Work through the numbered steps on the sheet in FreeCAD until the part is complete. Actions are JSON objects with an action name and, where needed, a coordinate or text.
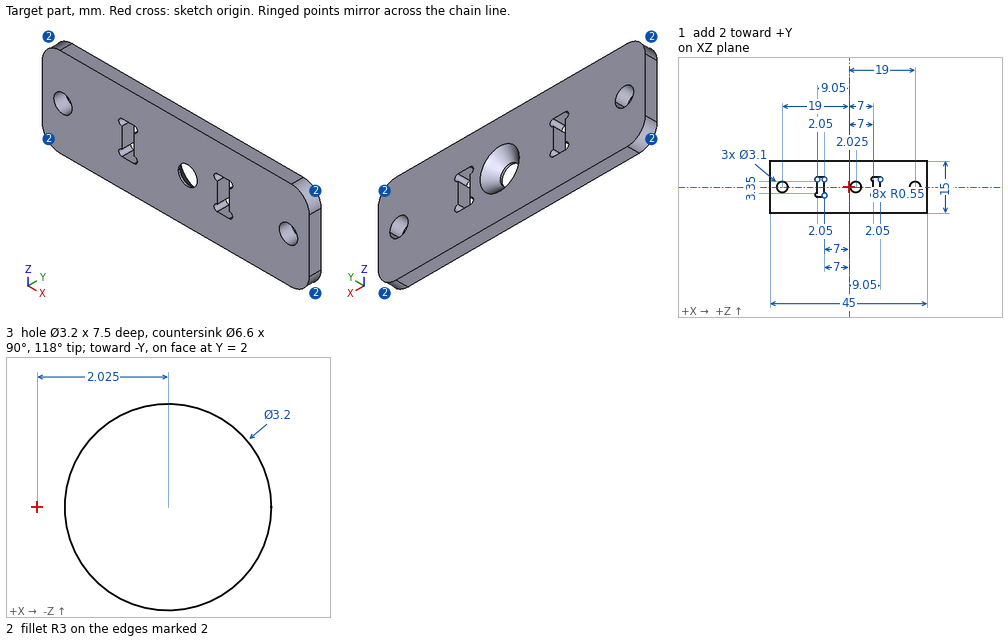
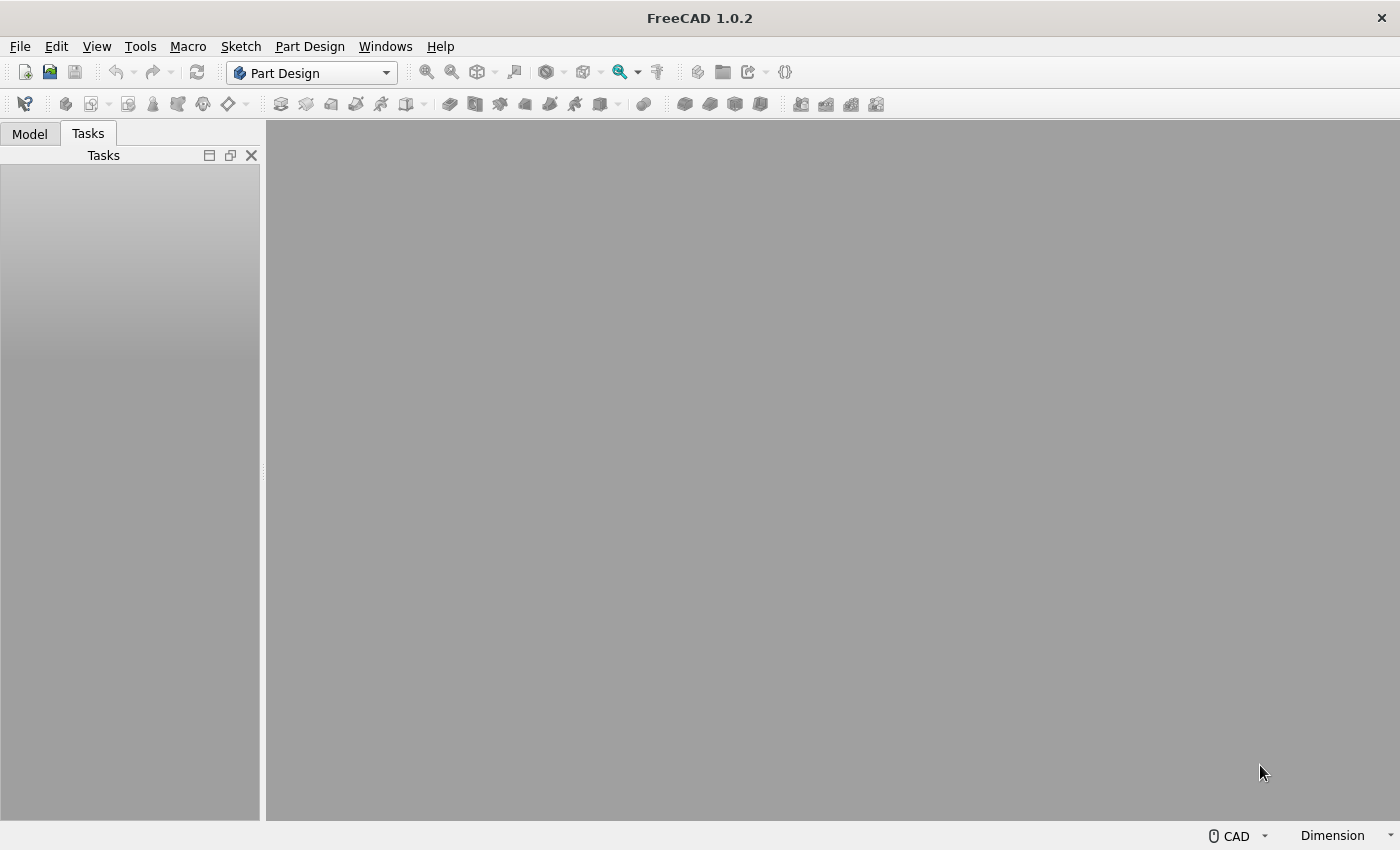
{"action": "left_click", "coordinate": [25, 72]}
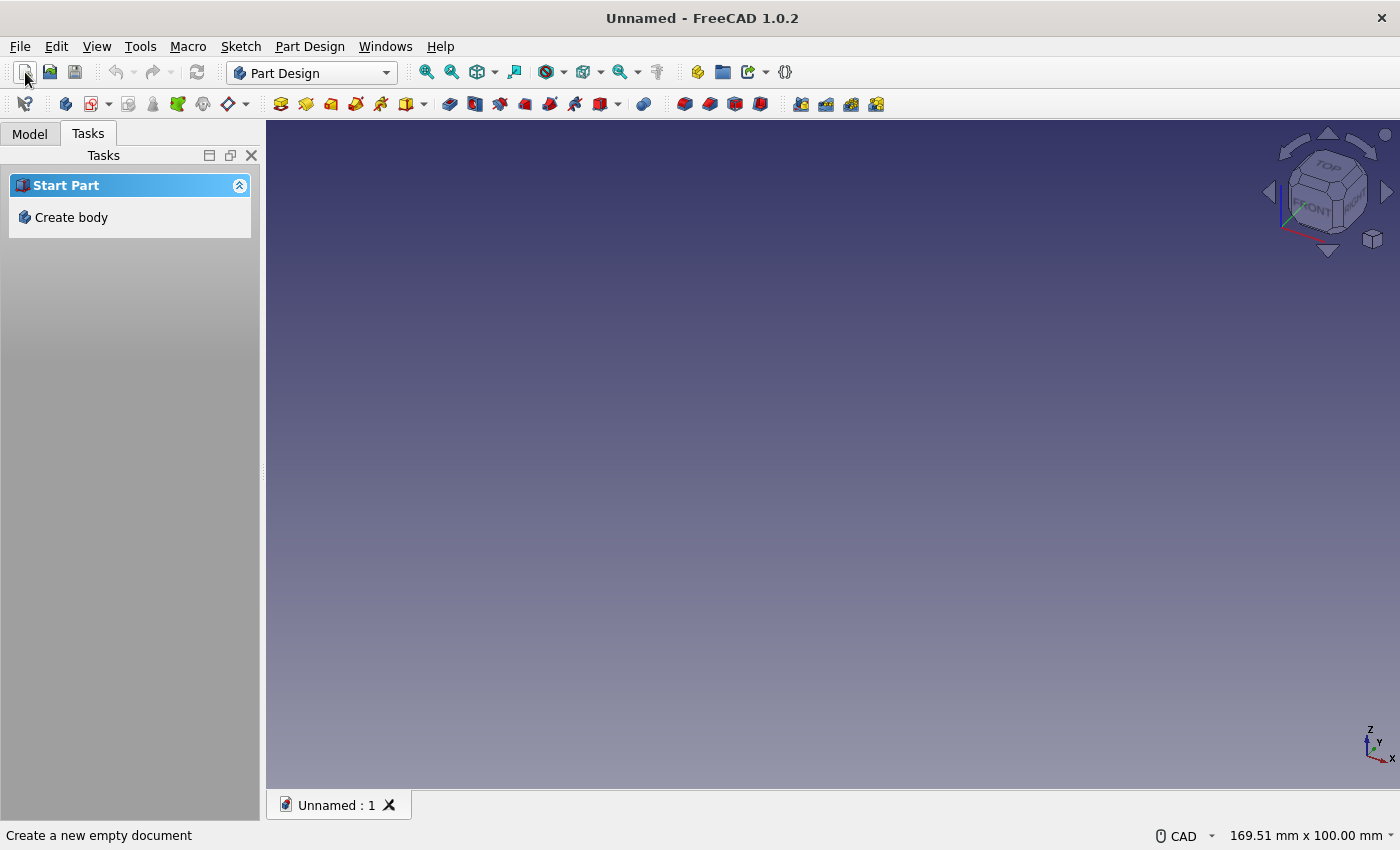
{"action": "left_click", "coordinate": [90, 104]}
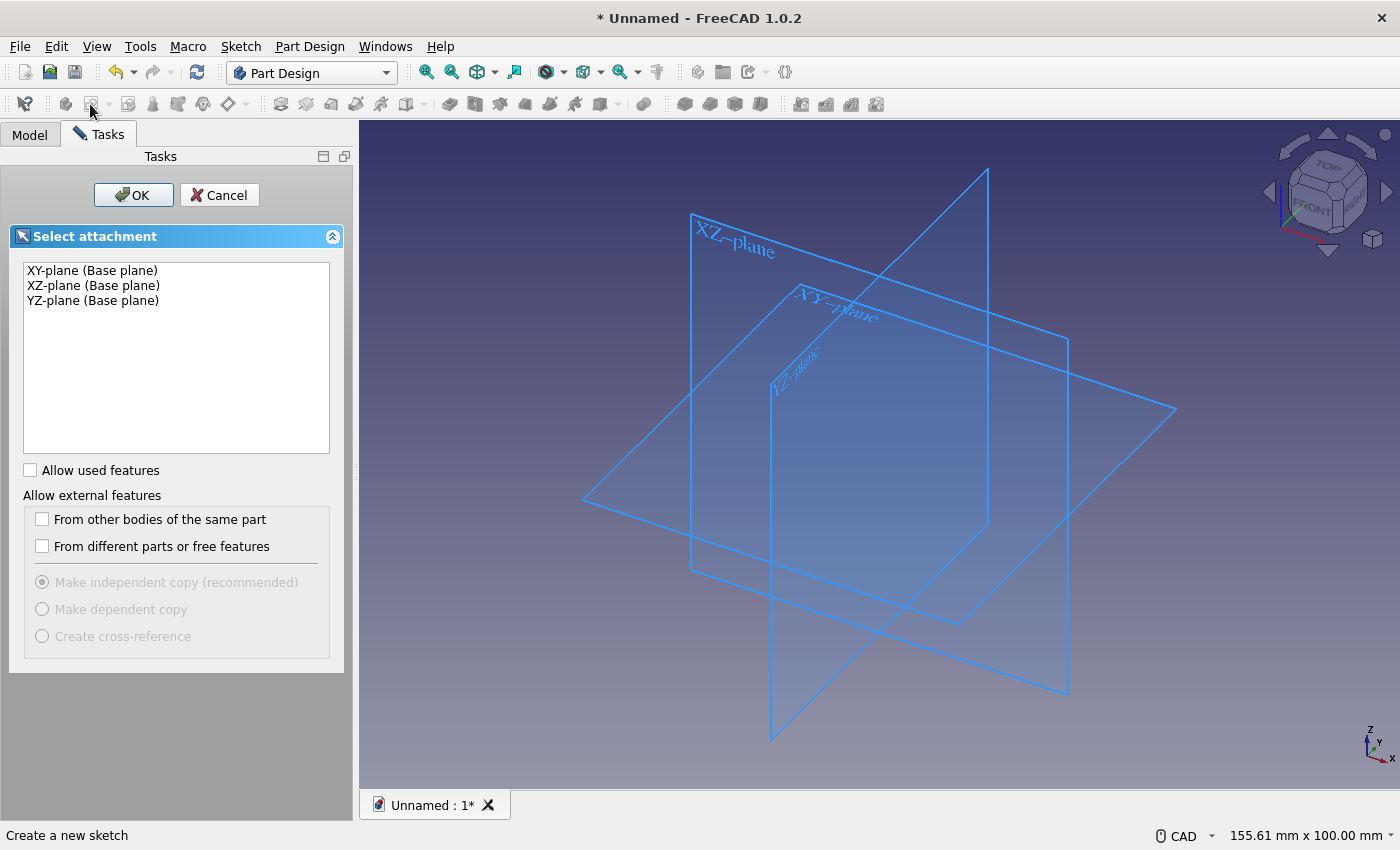
{"action": "left_click", "coordinate": [84, 286]}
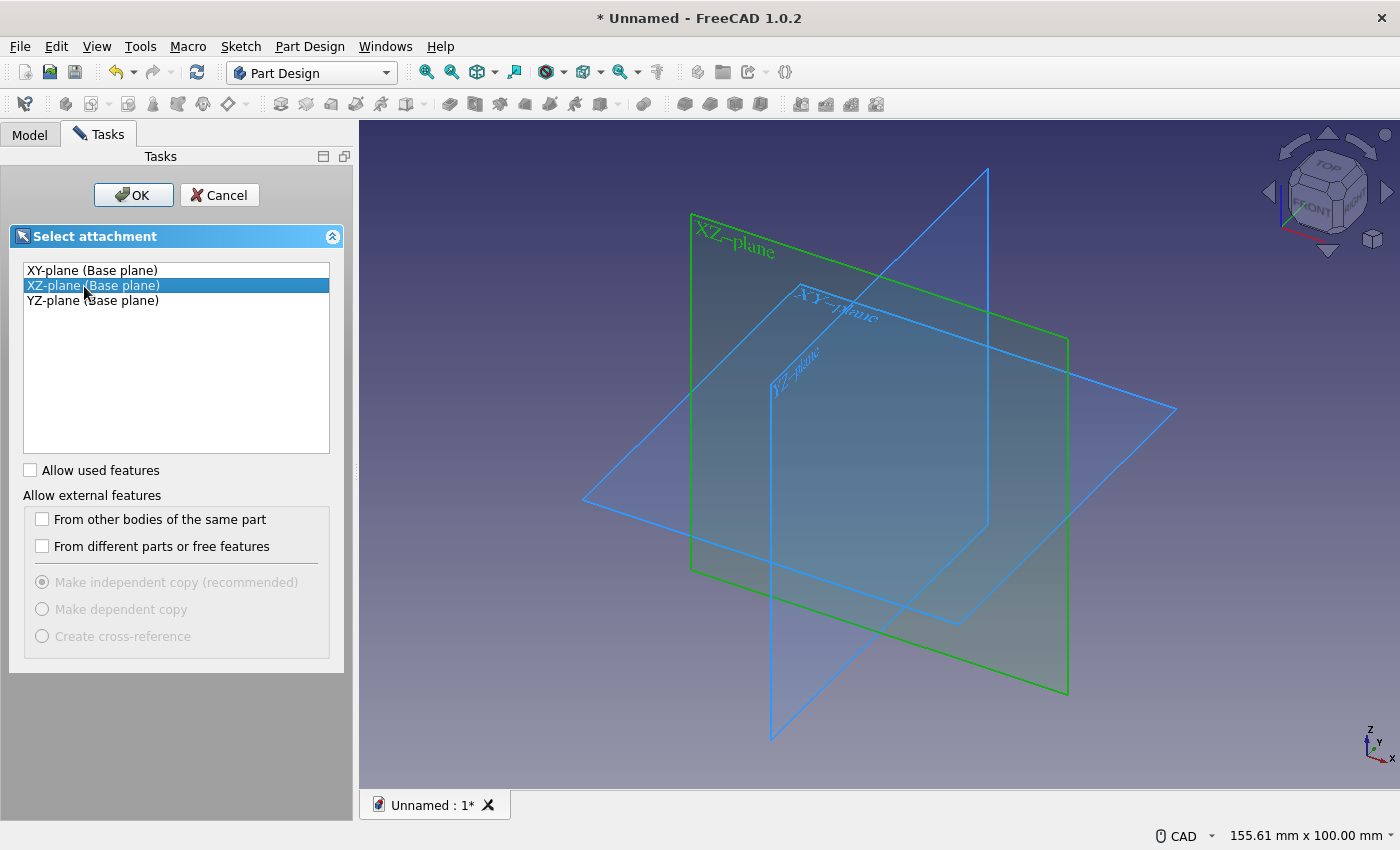
{"action": "left_click", "coordinate": [134, 195]}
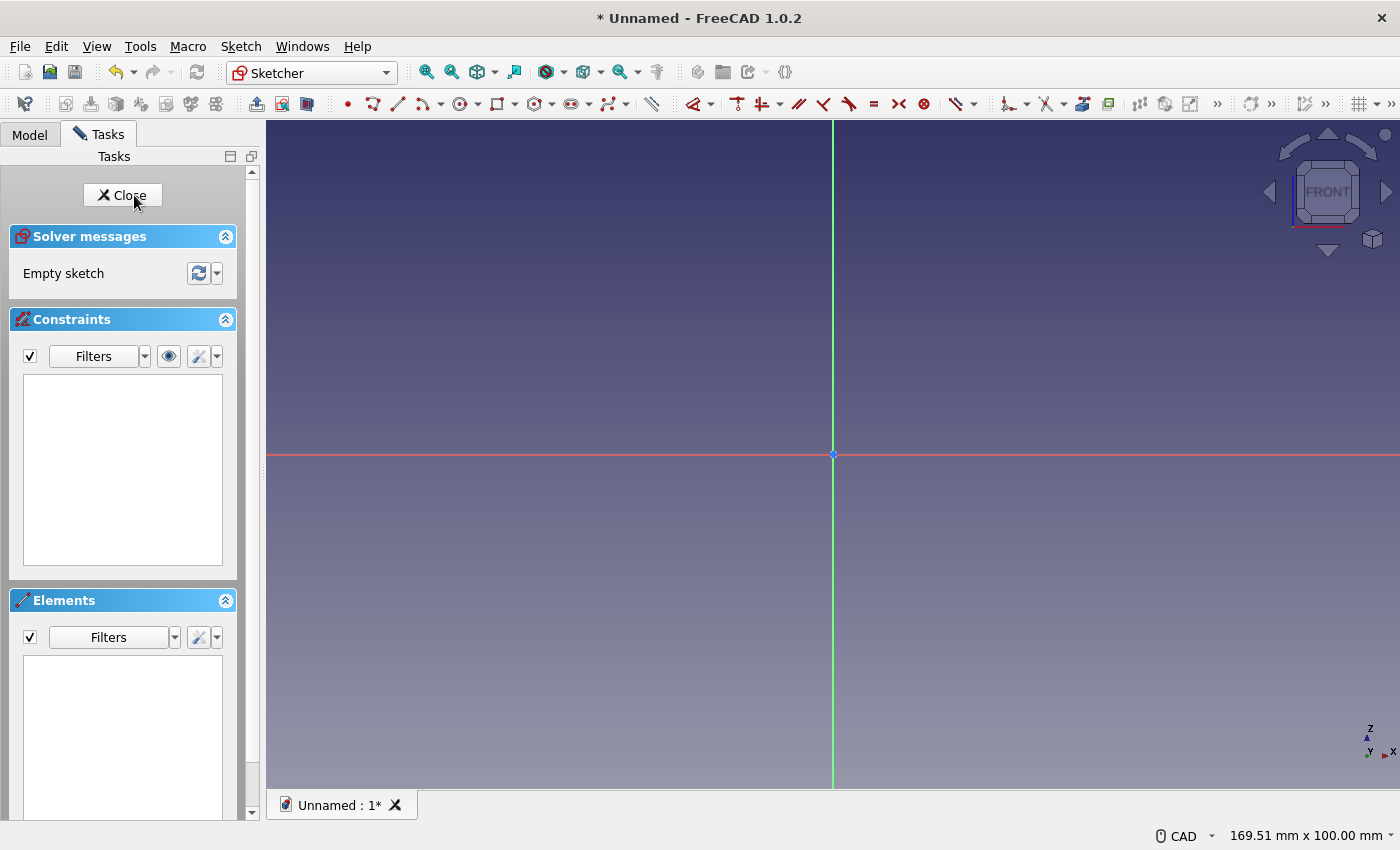
{"action": "scroll", "coordinate": [889, 455], "scroll_direction": "up", "scroll_amount": 4}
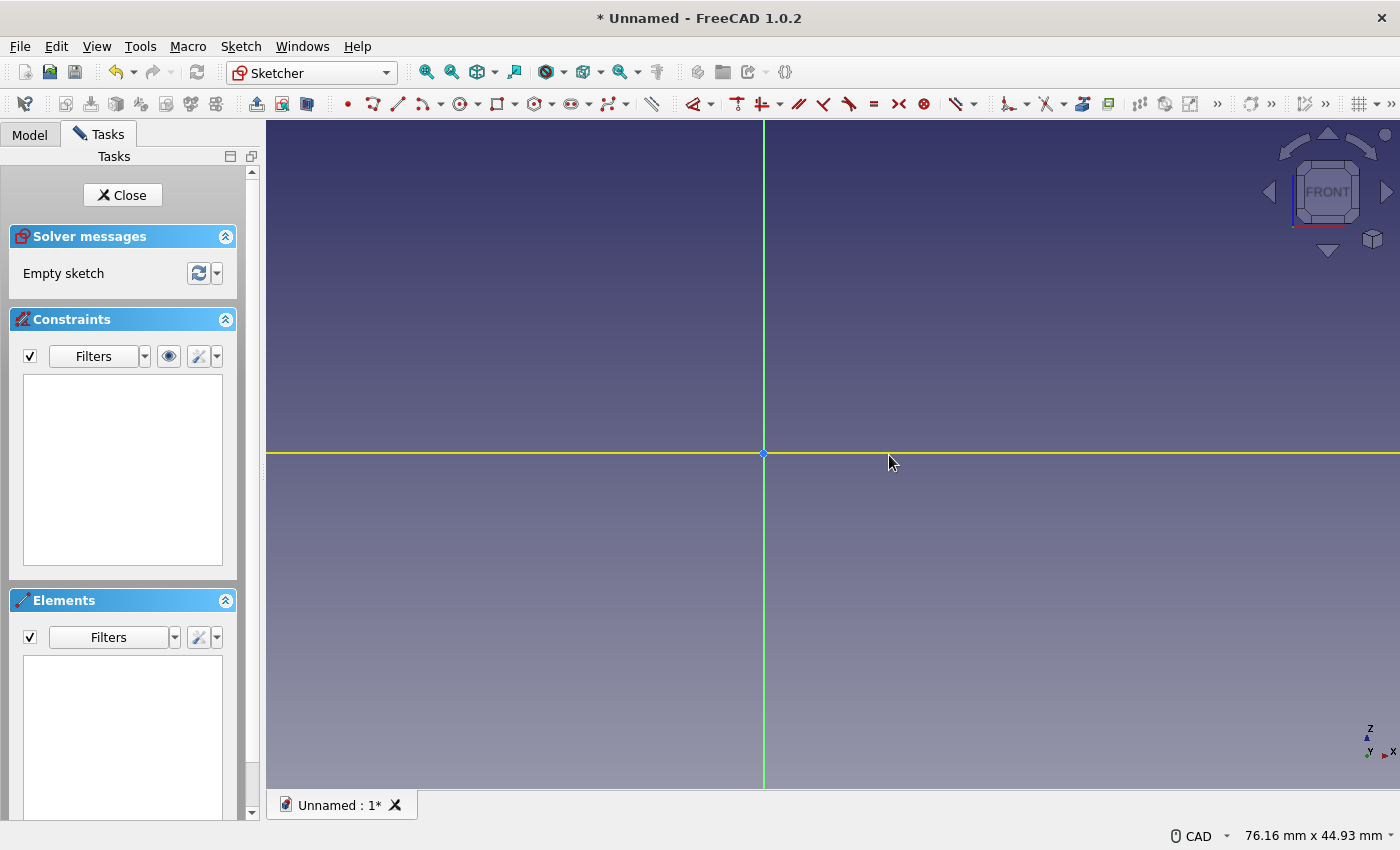
{"action": "key", "text": "g v"}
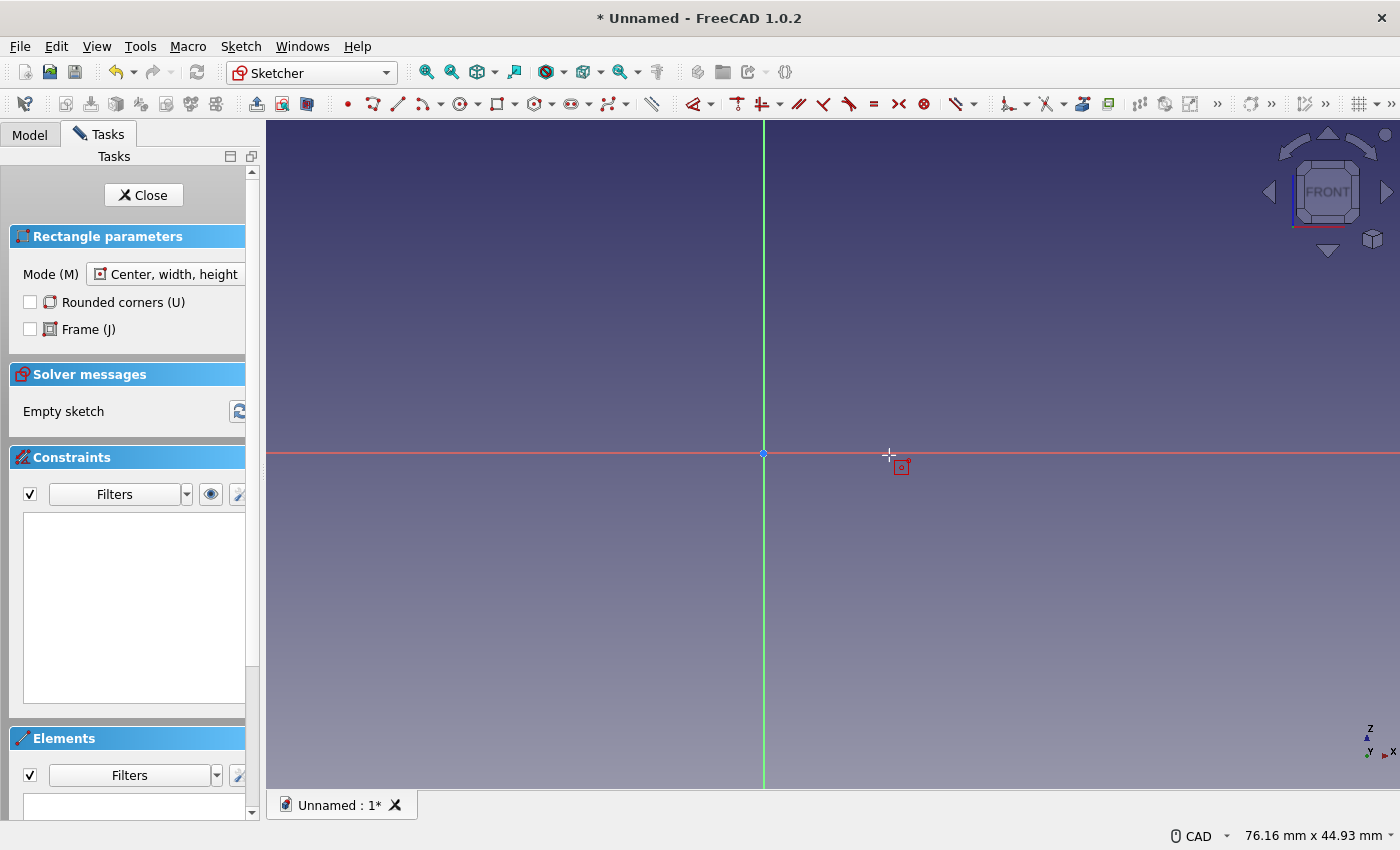
{"action": "left_click", "coordinate": [764, 453]}
{"action": "mouse_move", "coordinate": [1099, 342]}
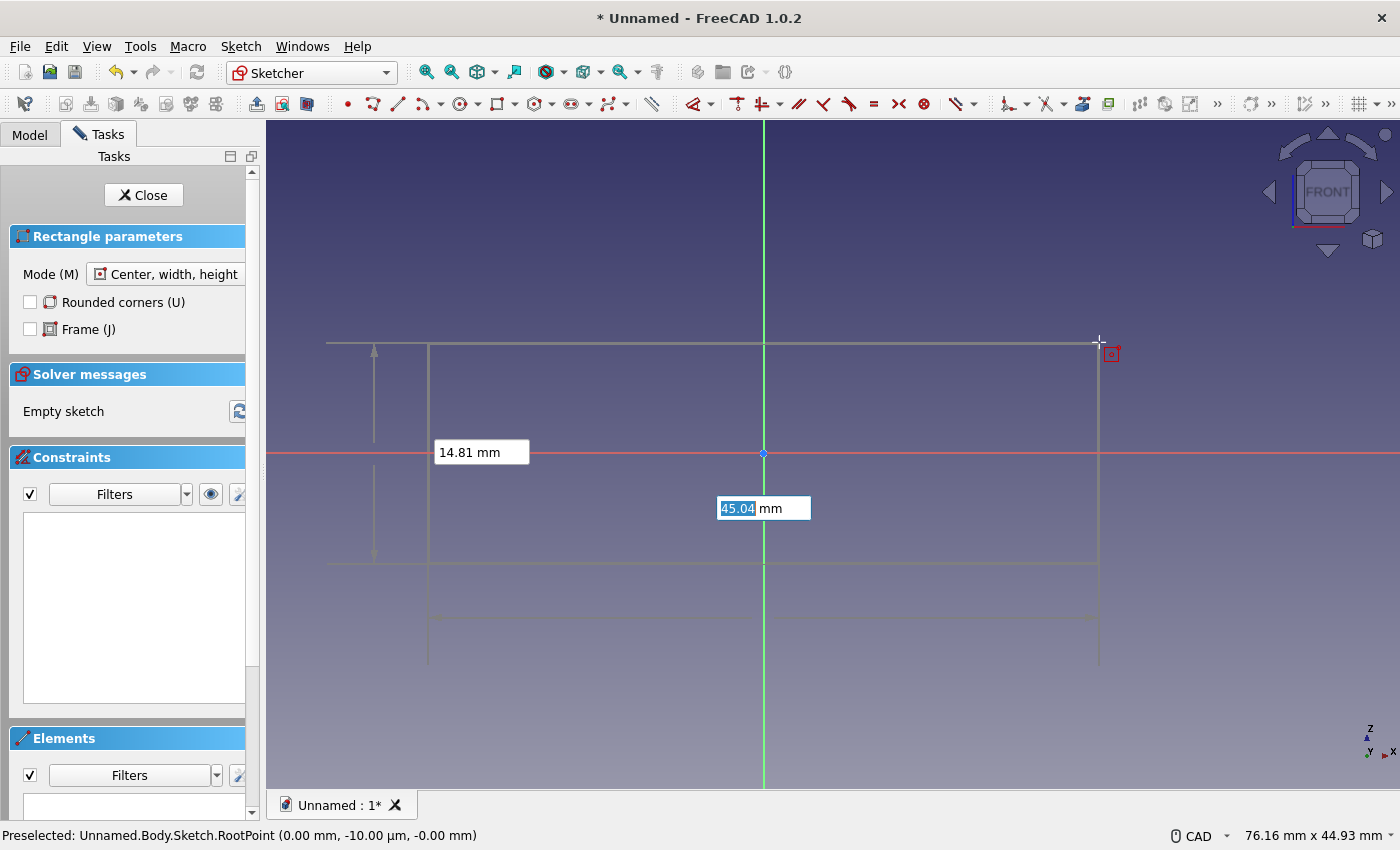
{"action": "type", "text": "45"}
{"action": "key", "text": "Tab"}
{"action": "type", "text": "15"}
{"action": "key", "text": "Return"}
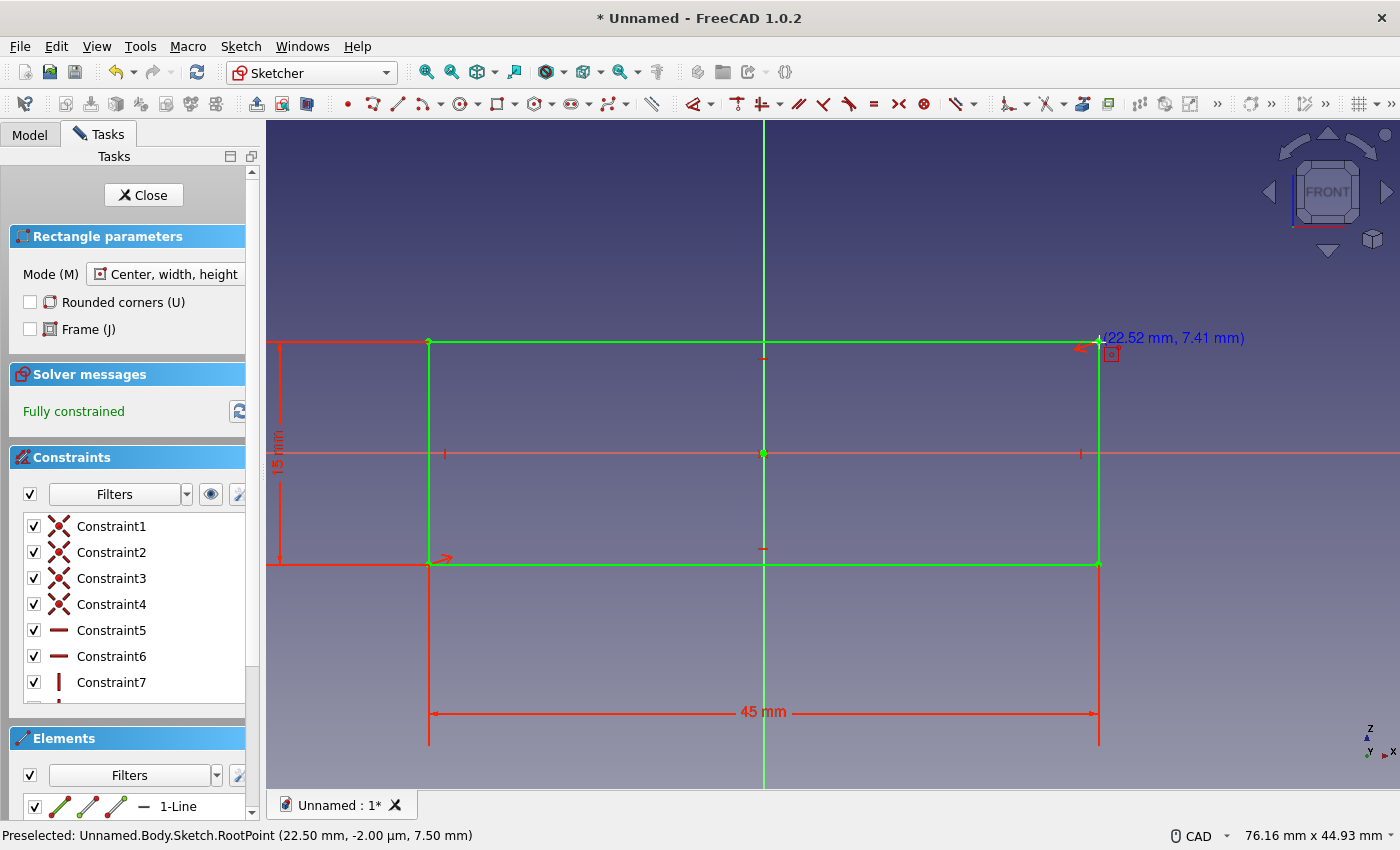
{"action": "left_click", "coordinate": [398, 104]}